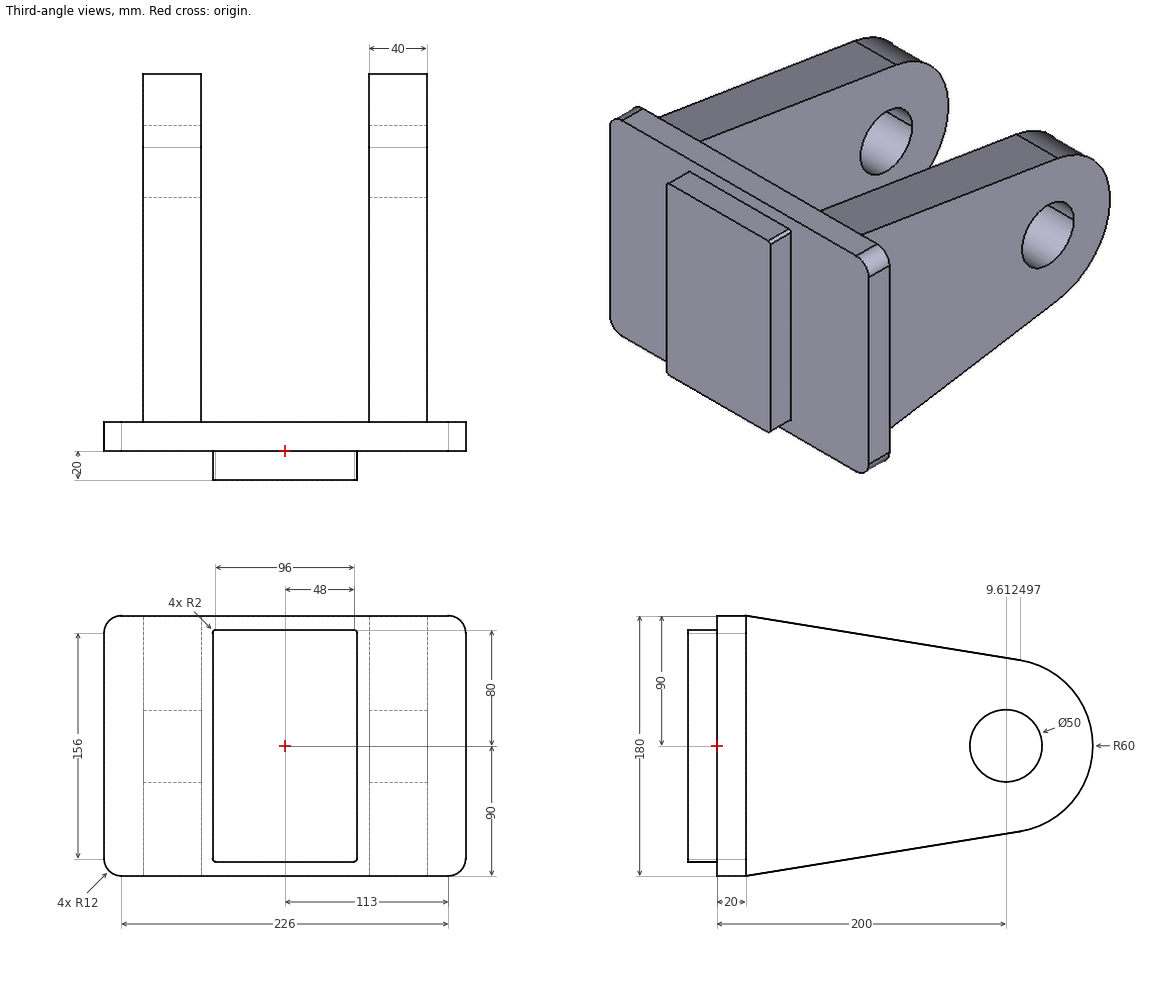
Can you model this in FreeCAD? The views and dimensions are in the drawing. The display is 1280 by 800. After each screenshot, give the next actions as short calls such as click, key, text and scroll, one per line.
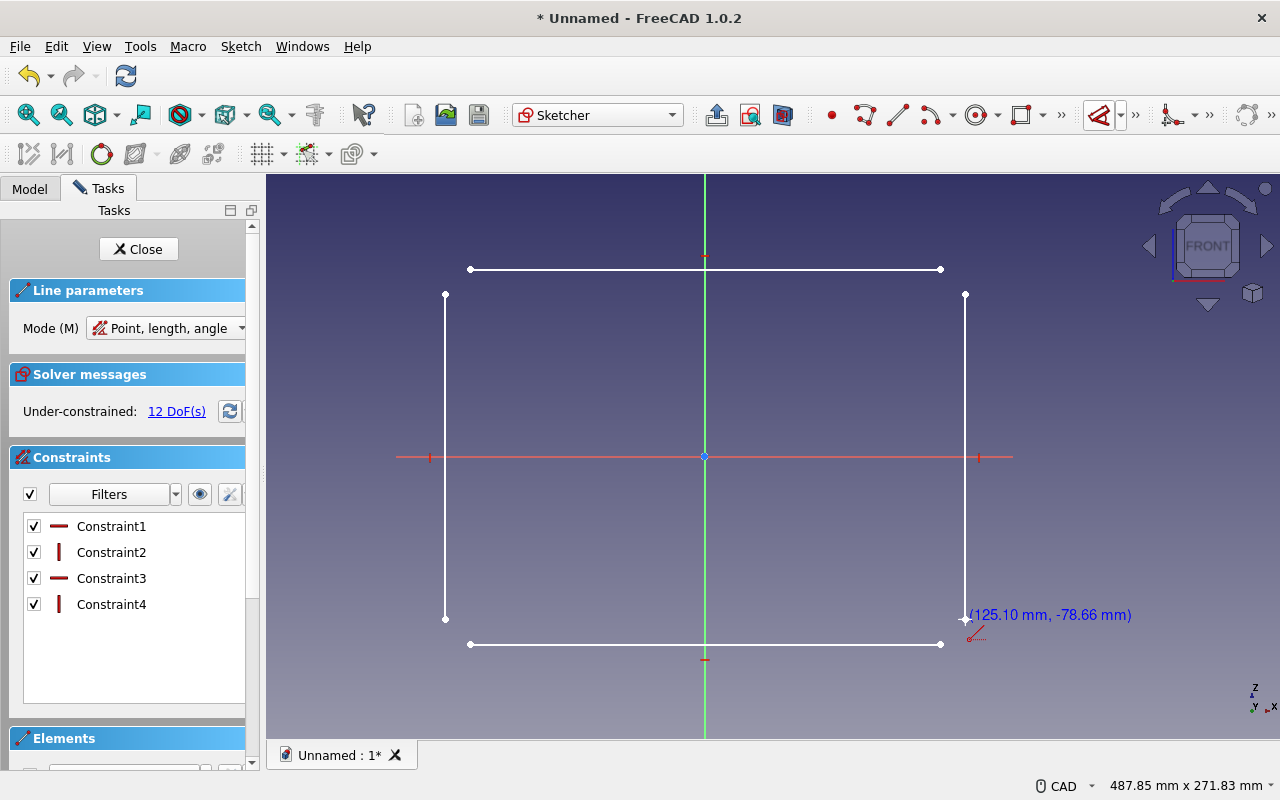
click(952, 116)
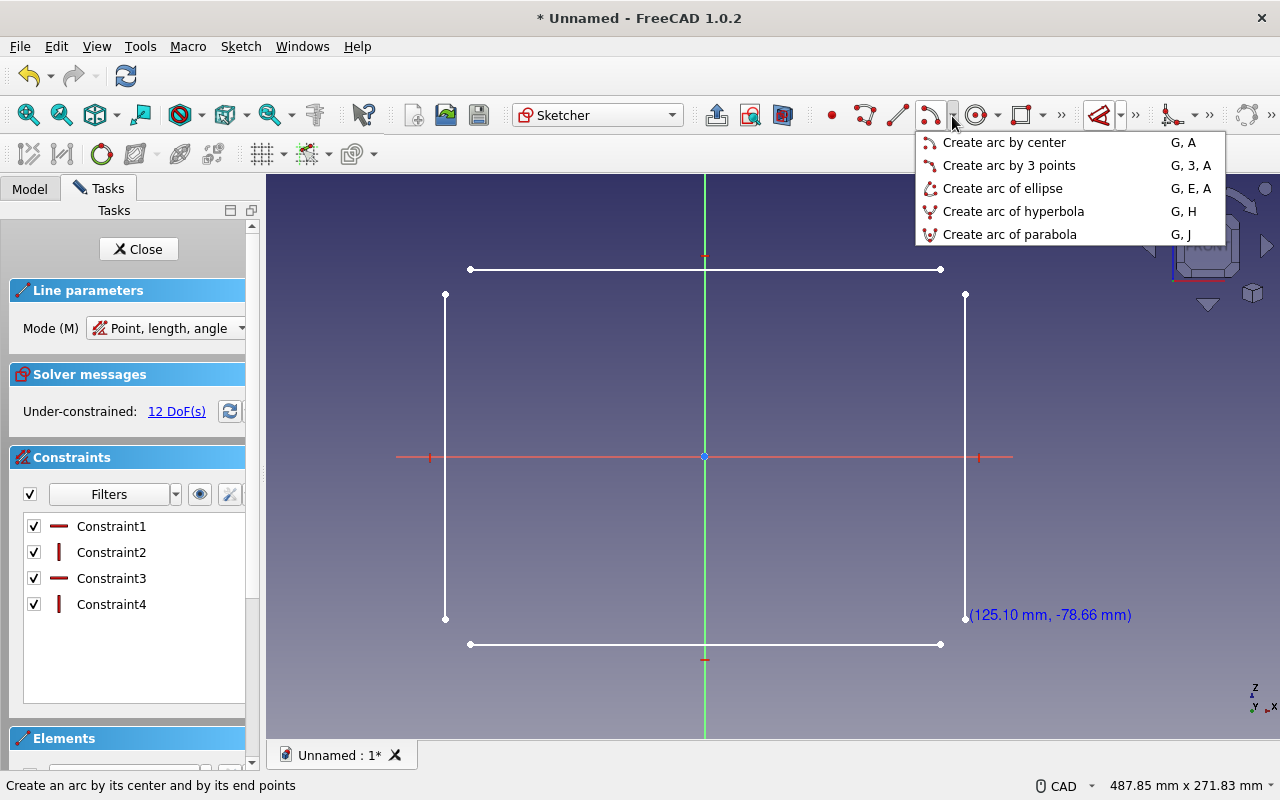
click(1070, 166)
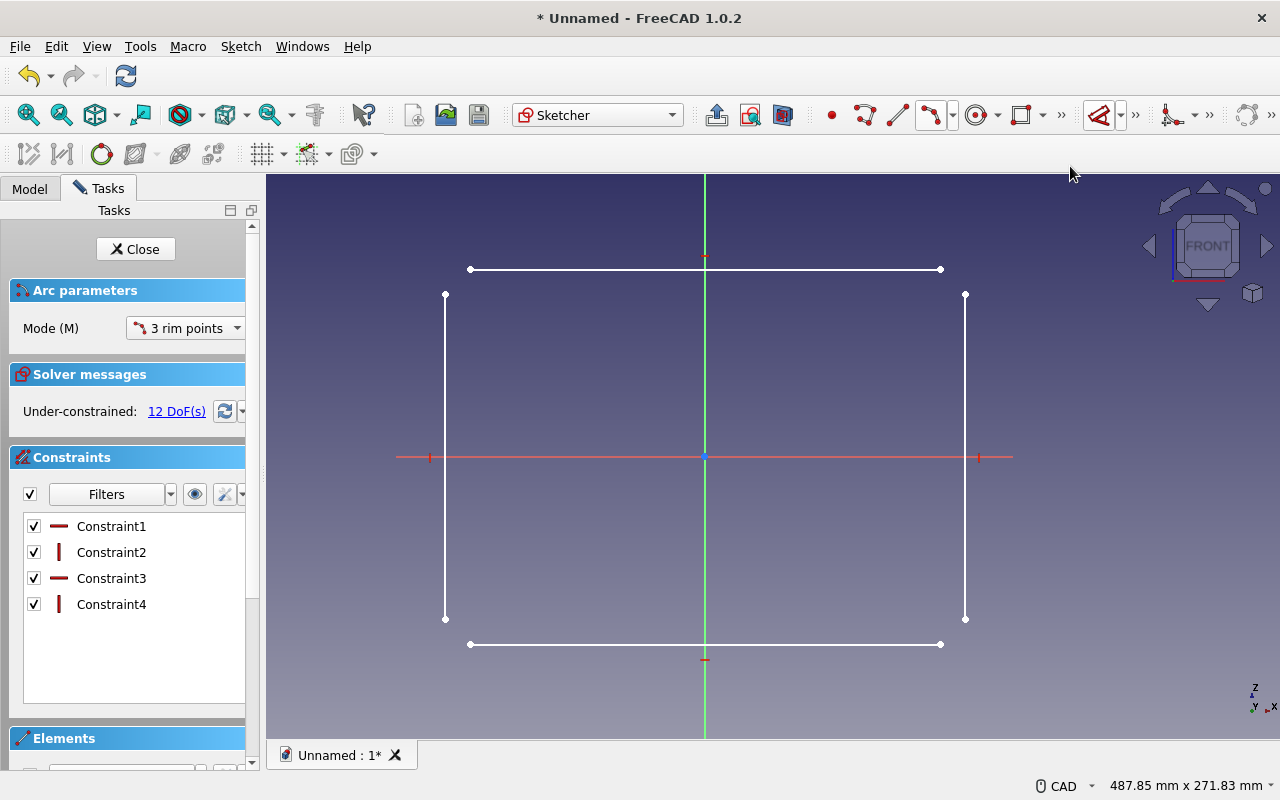
click(470, 645)
click(445, 620)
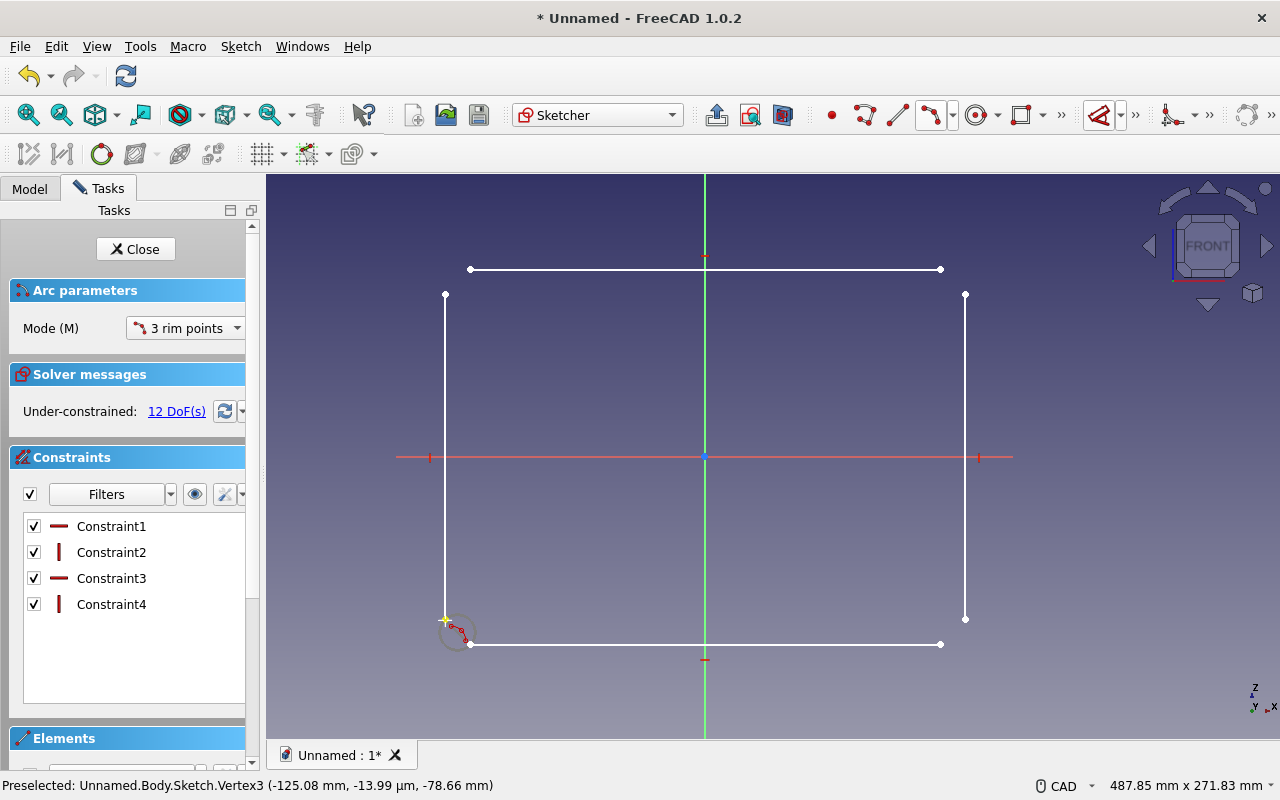
scroll(452, 636, up, 4)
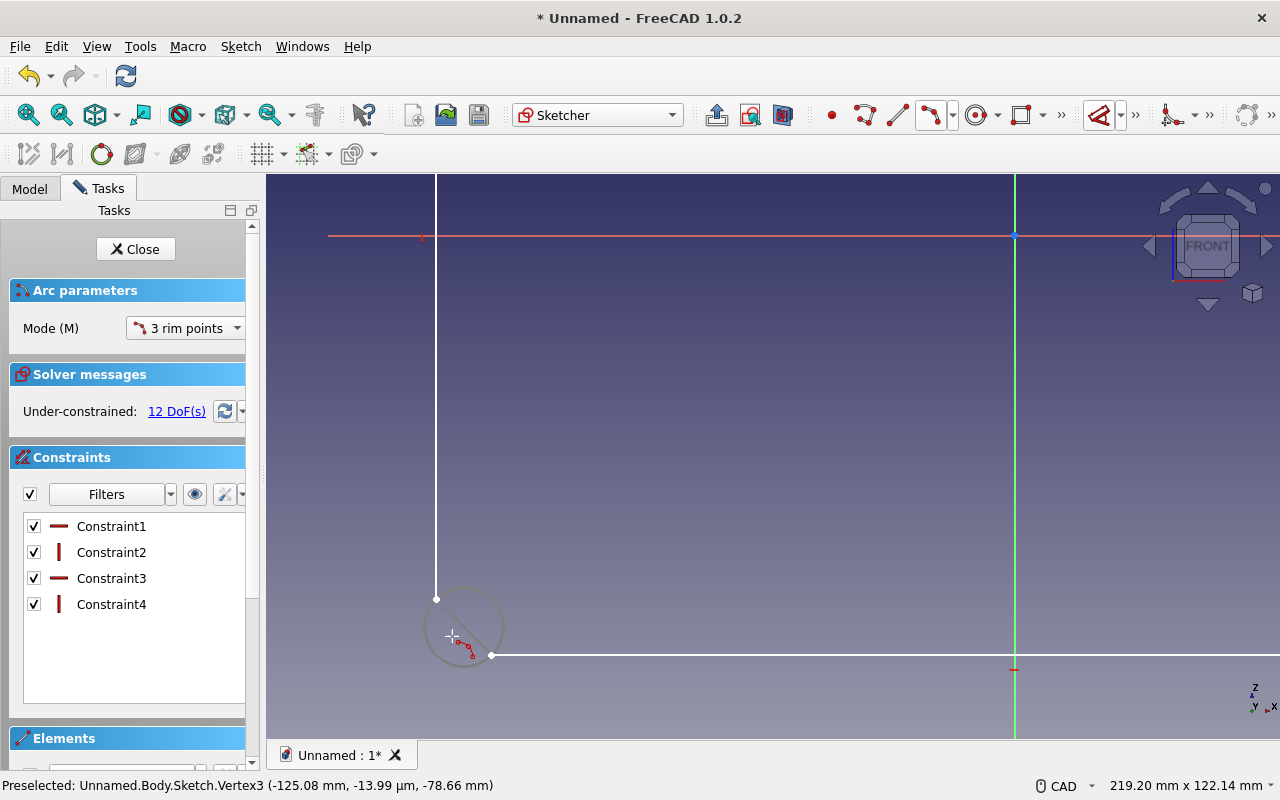
click(453, 636)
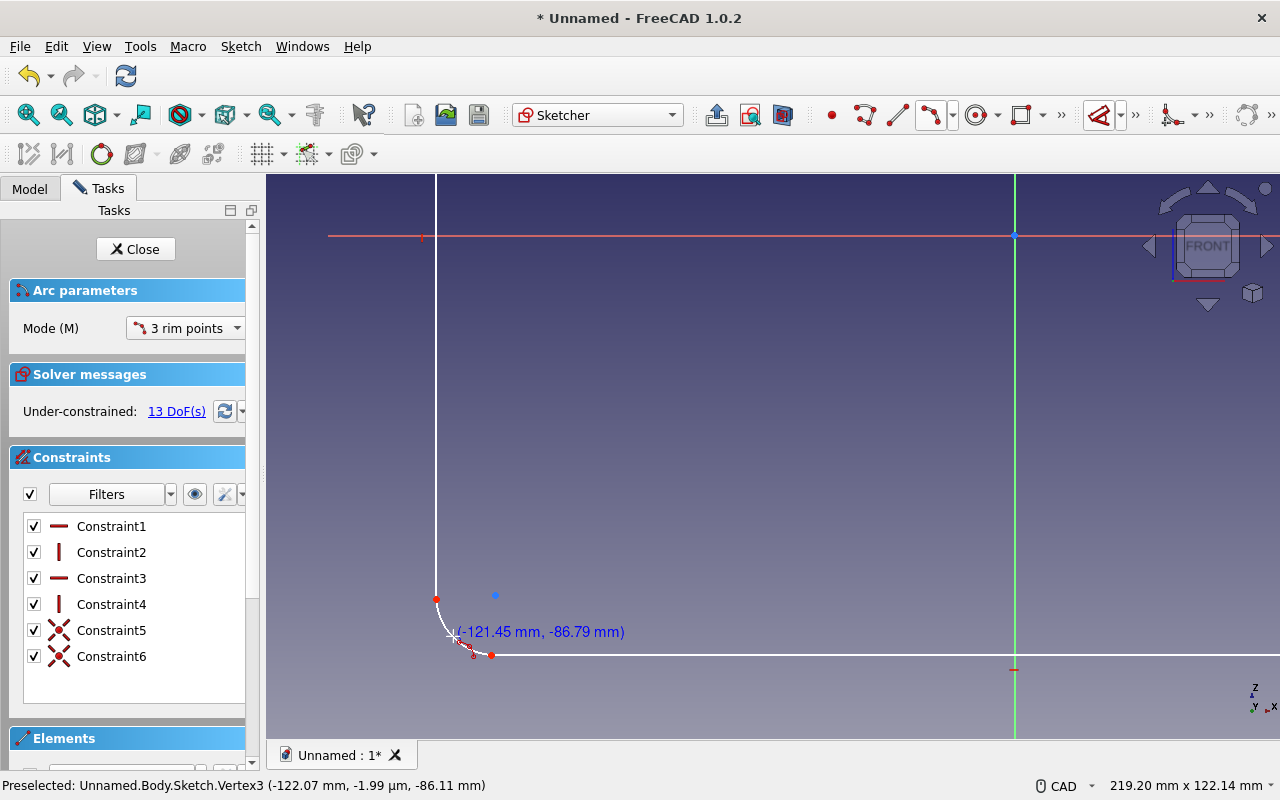
scroll(451, 637, down, 4)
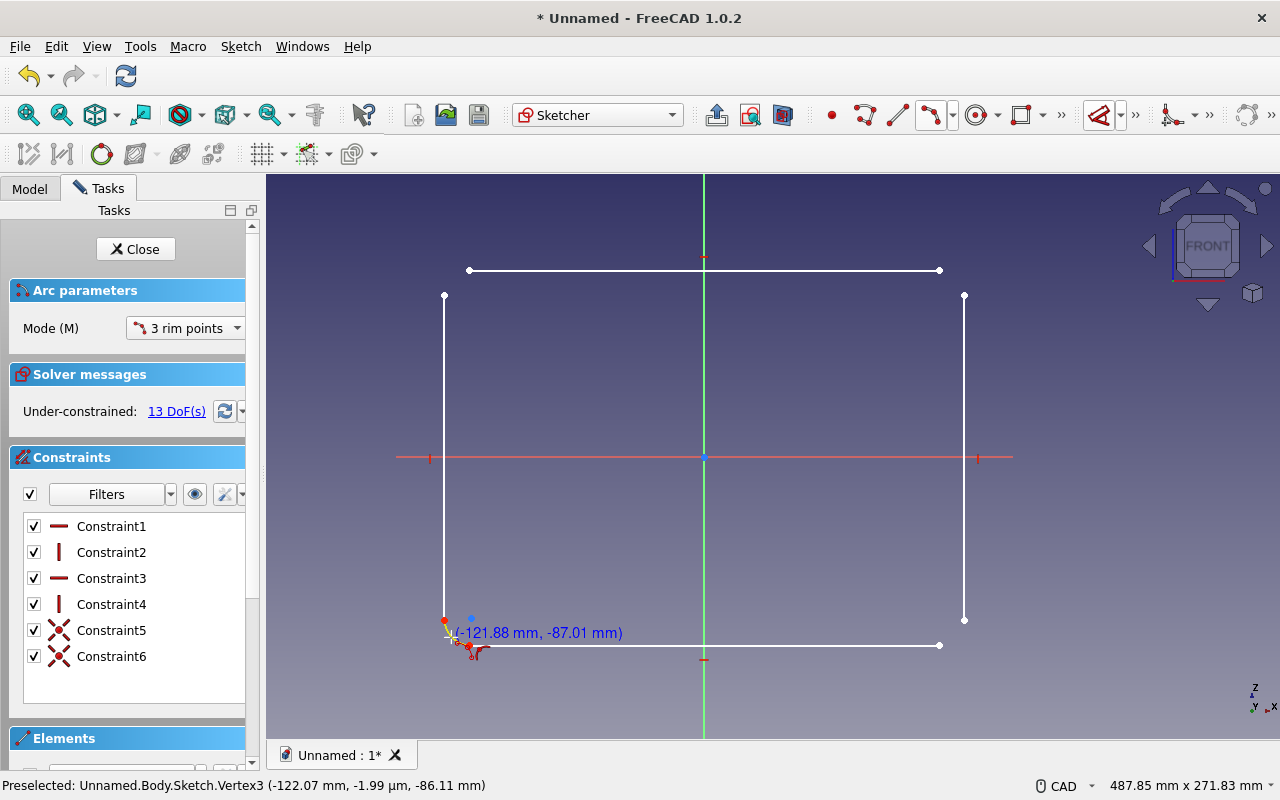
click(444, 296)
click(469, 271)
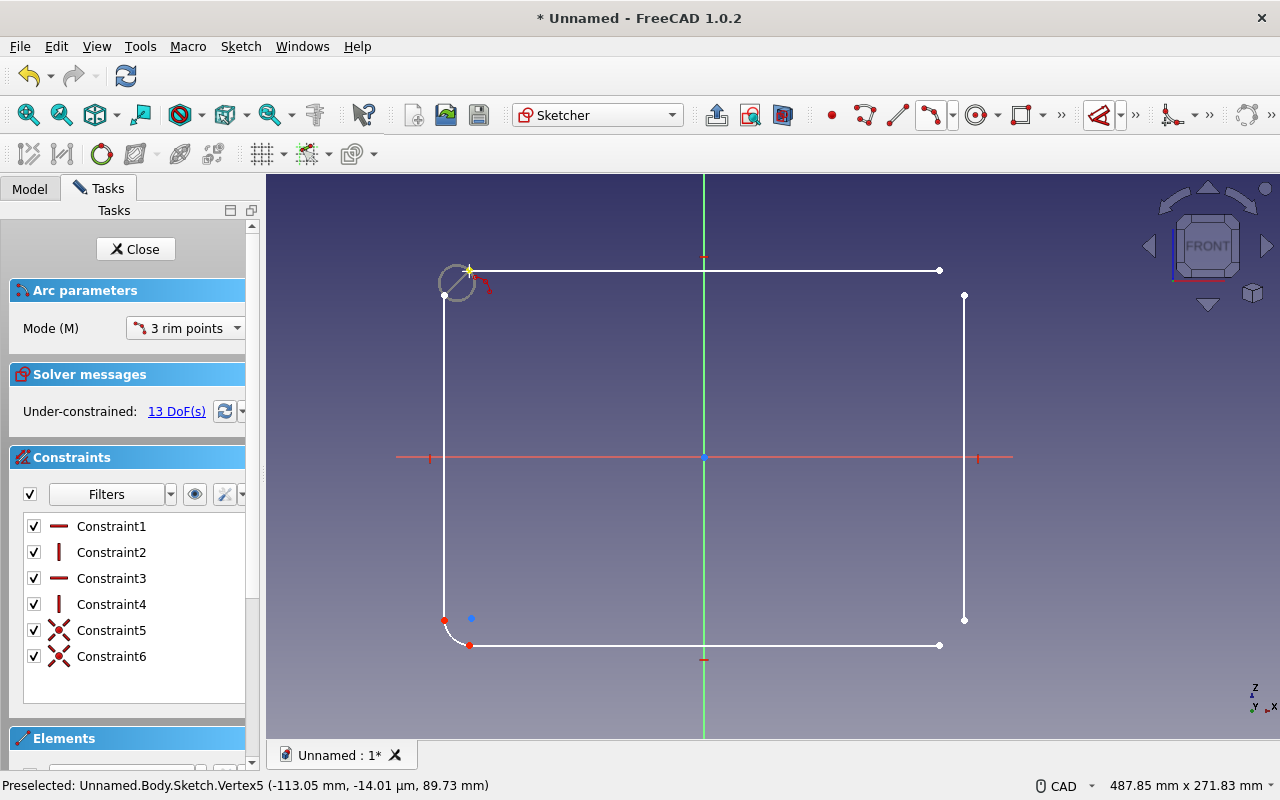
scroll(452, 277, up, 4)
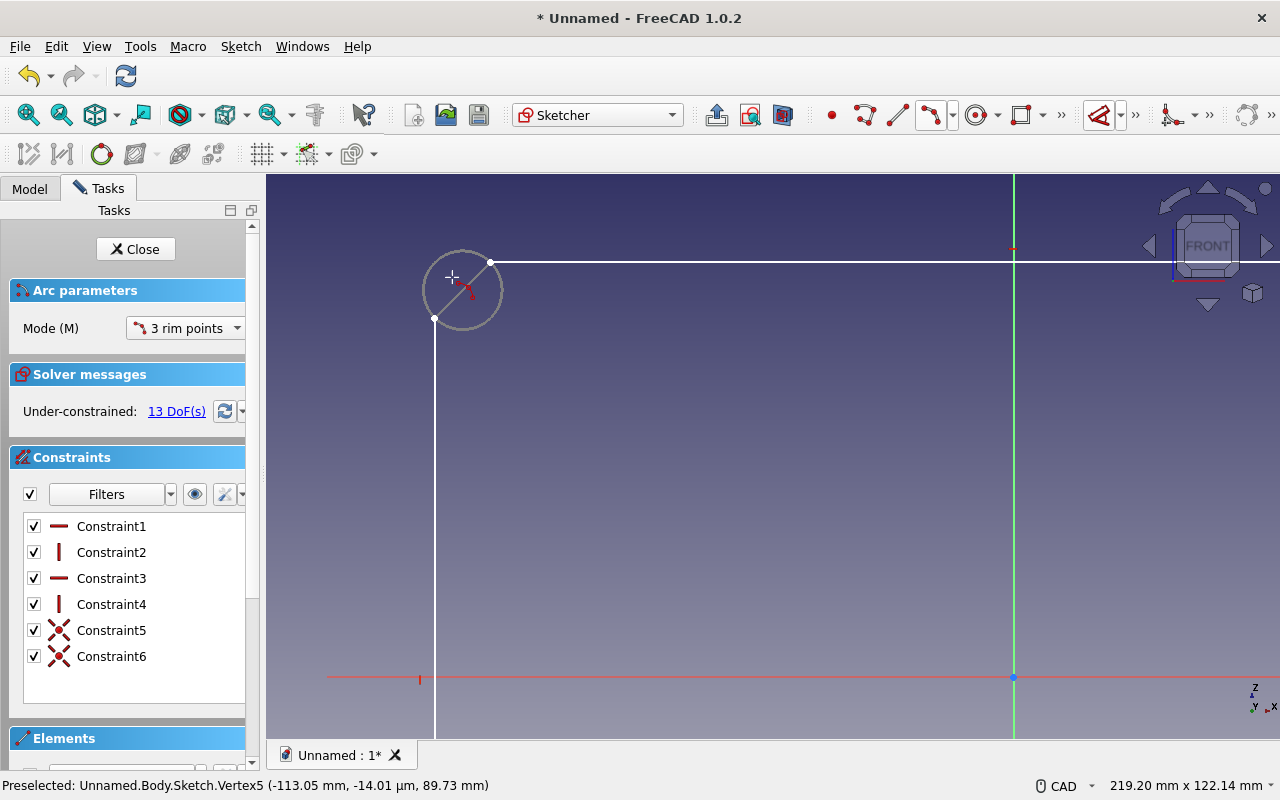
click(452, 277)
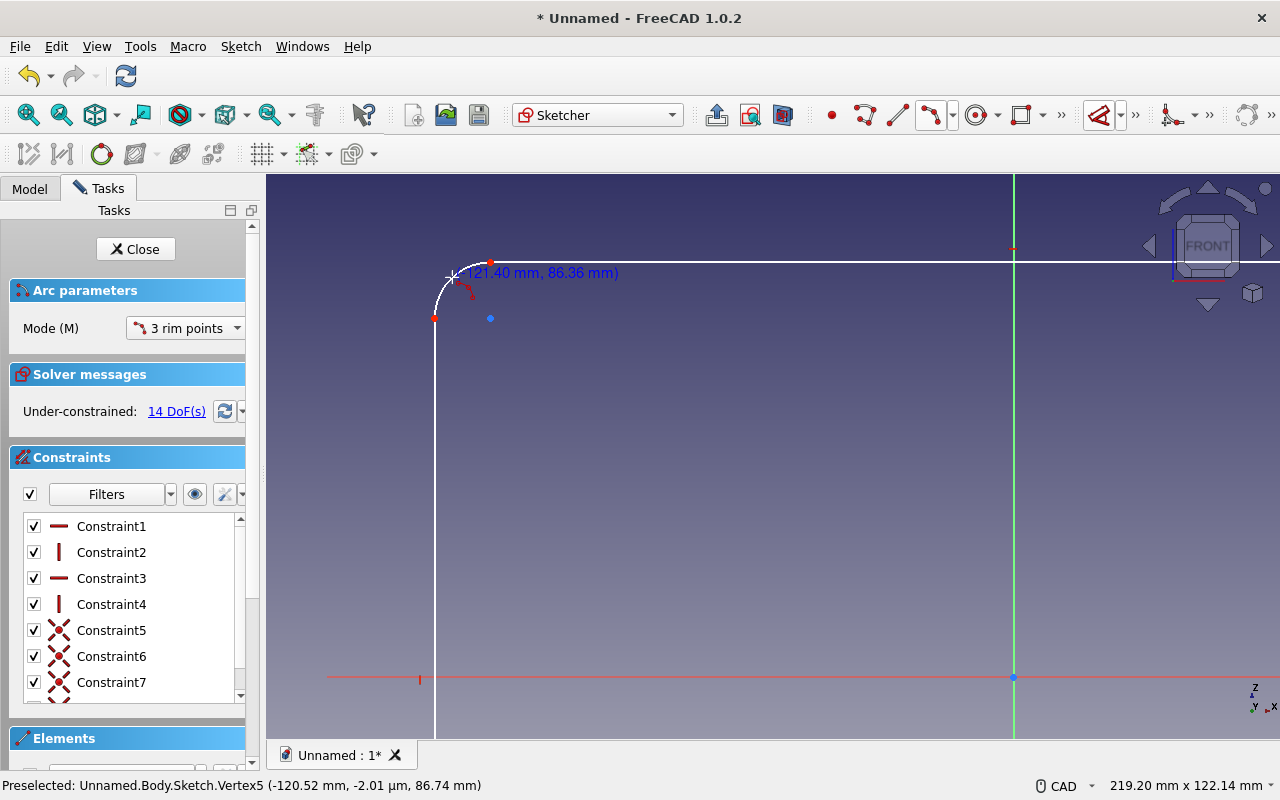
scroll(452, 276, down, 4)